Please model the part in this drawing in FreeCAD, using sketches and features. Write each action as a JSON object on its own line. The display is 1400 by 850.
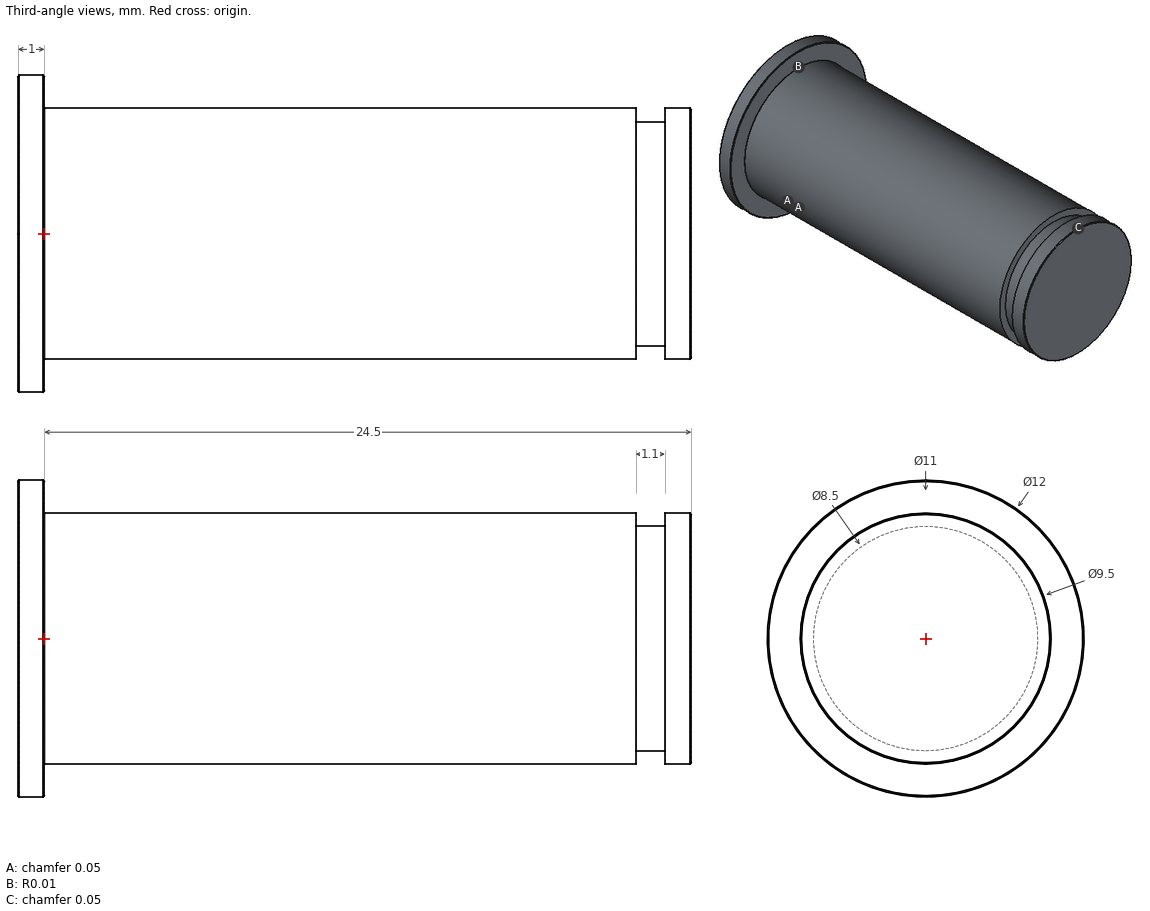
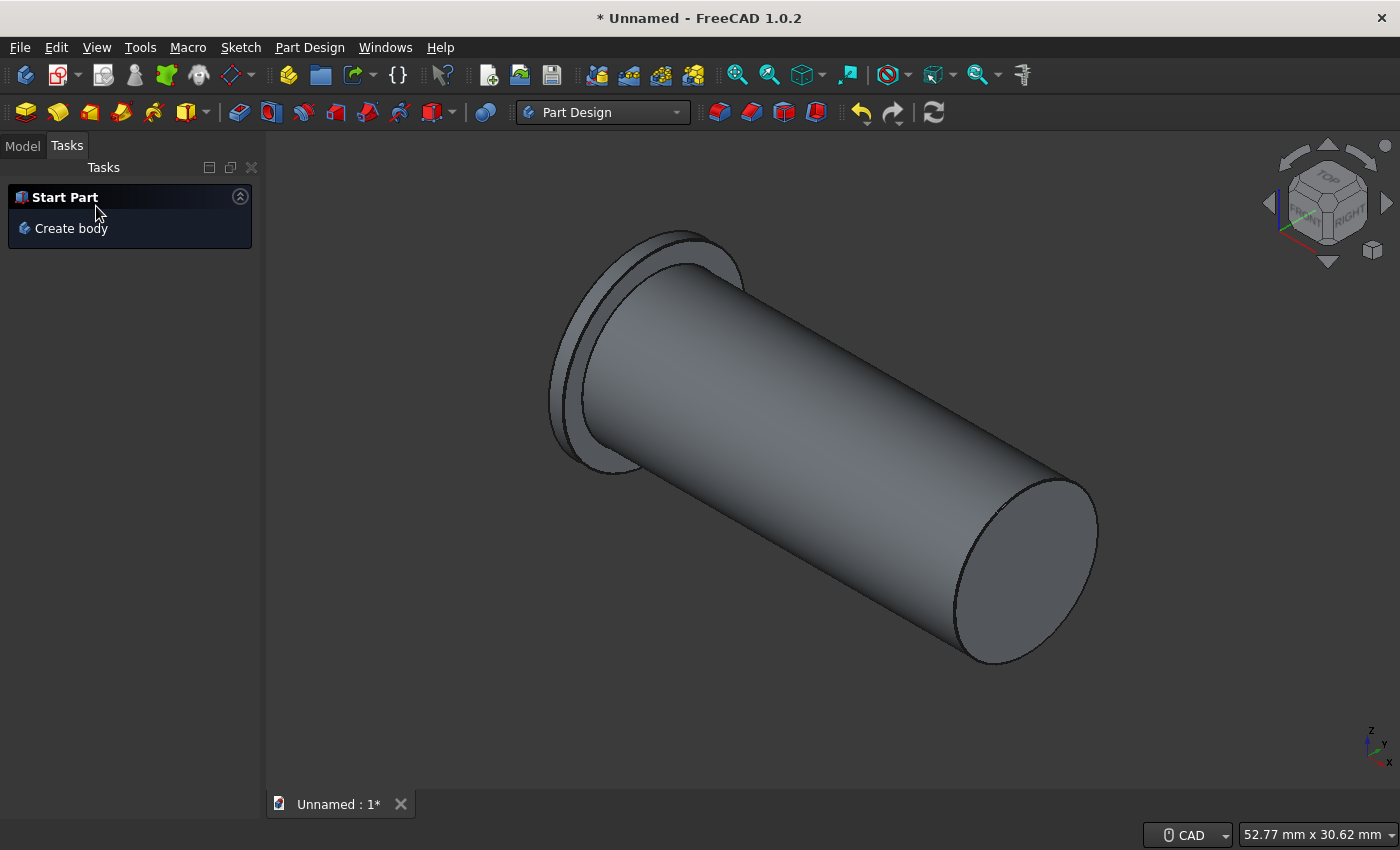
{"action": "left_click", "coordinate": [23, 145]}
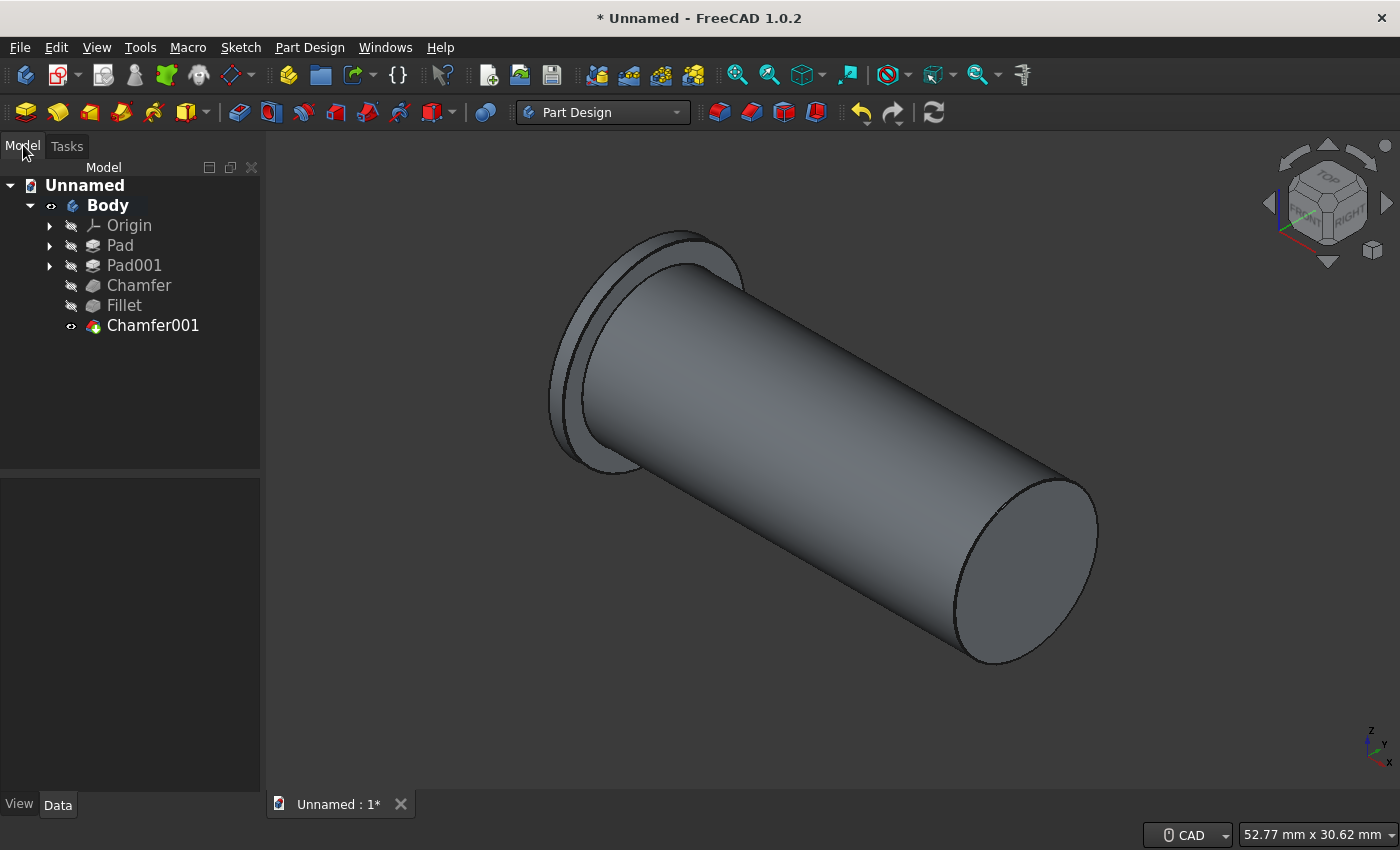
{"action": "left_click", "coordinate": [50, 226]}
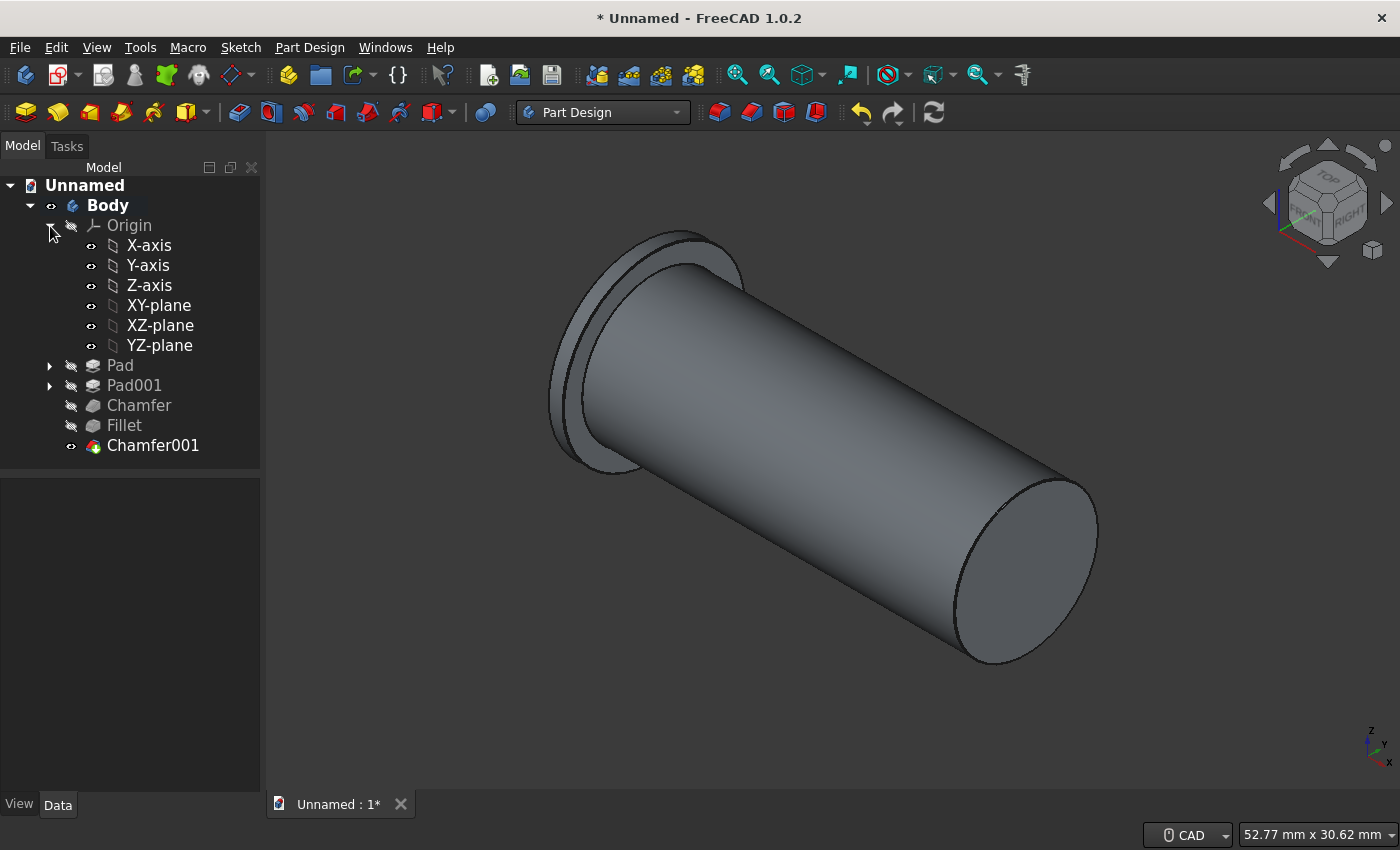
{"action": "left_click", "coordinate": [136, 346]}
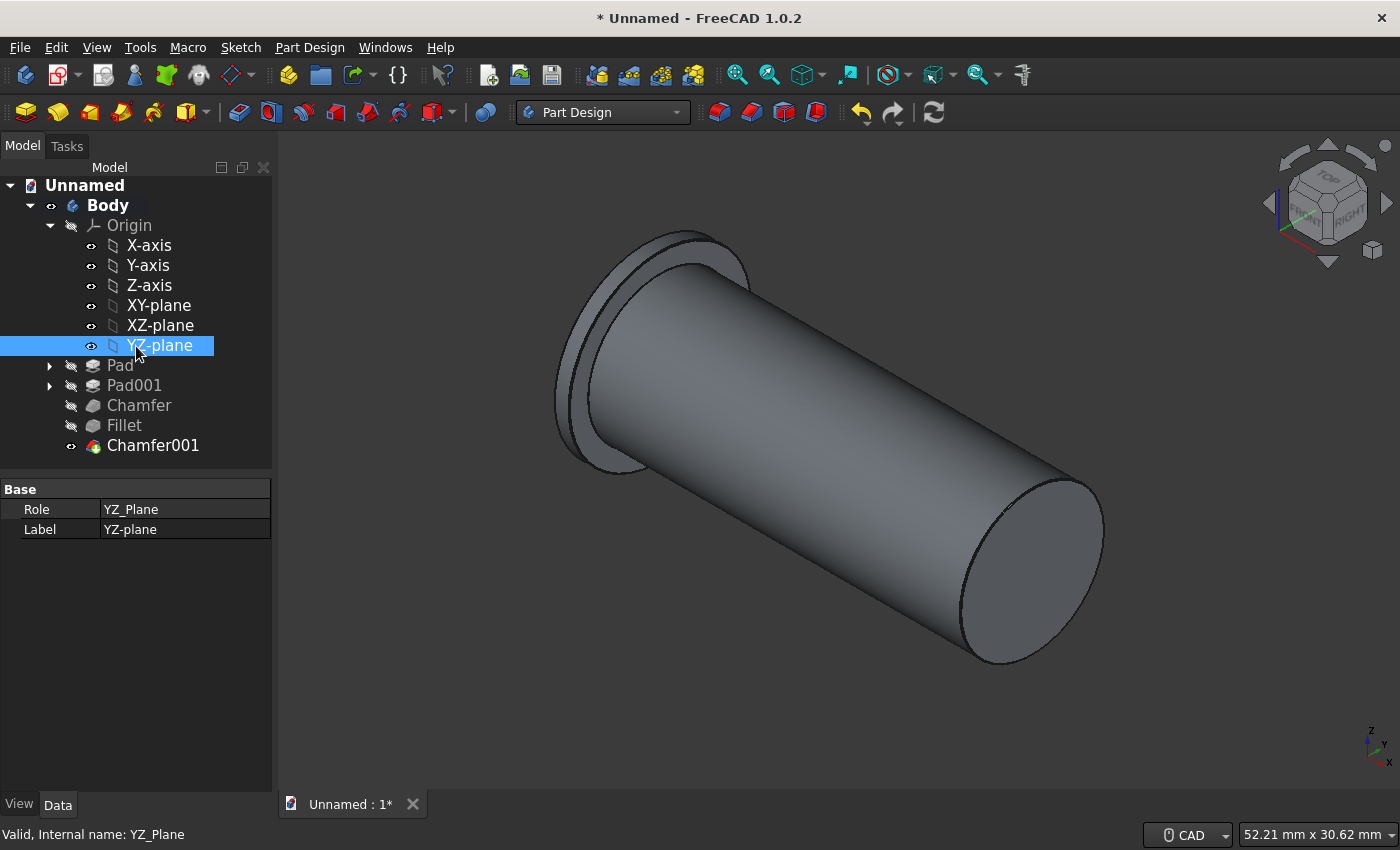
{"action": "left_click", "coordinate": [232, 76]}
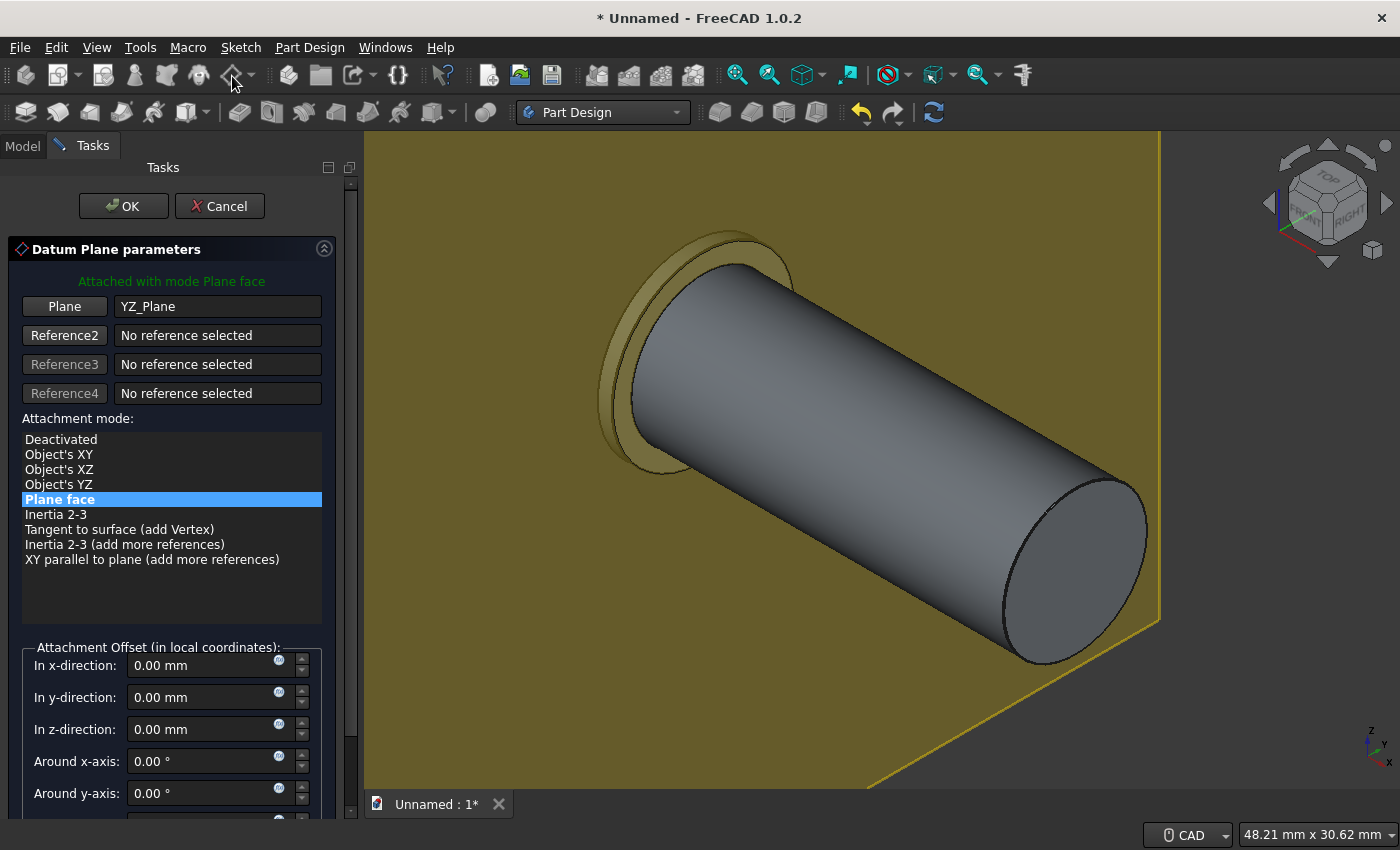
{"action": "triple_click", "coordinate": [210, 729]}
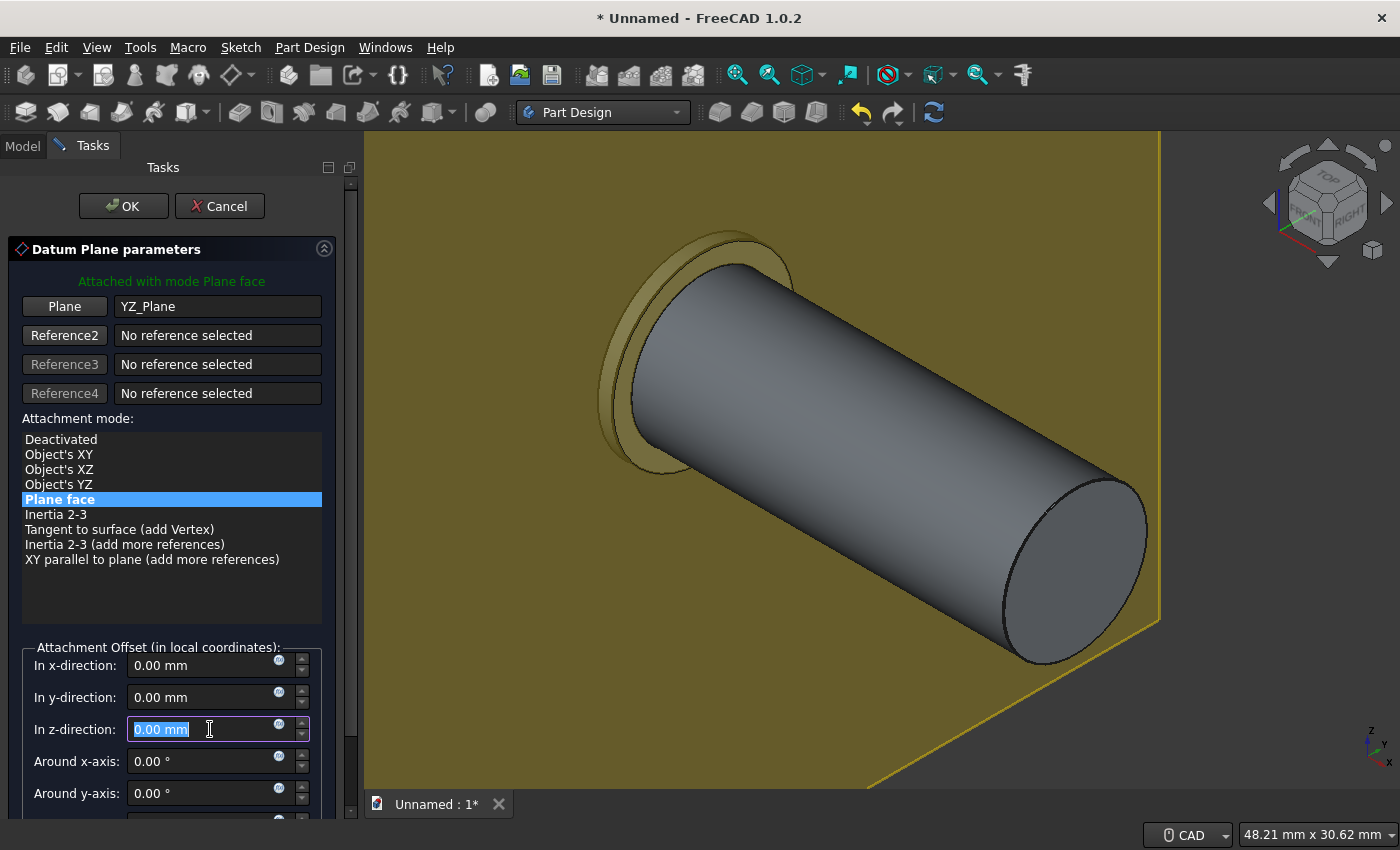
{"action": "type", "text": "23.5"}
{"action": "key", "text": "Tab"}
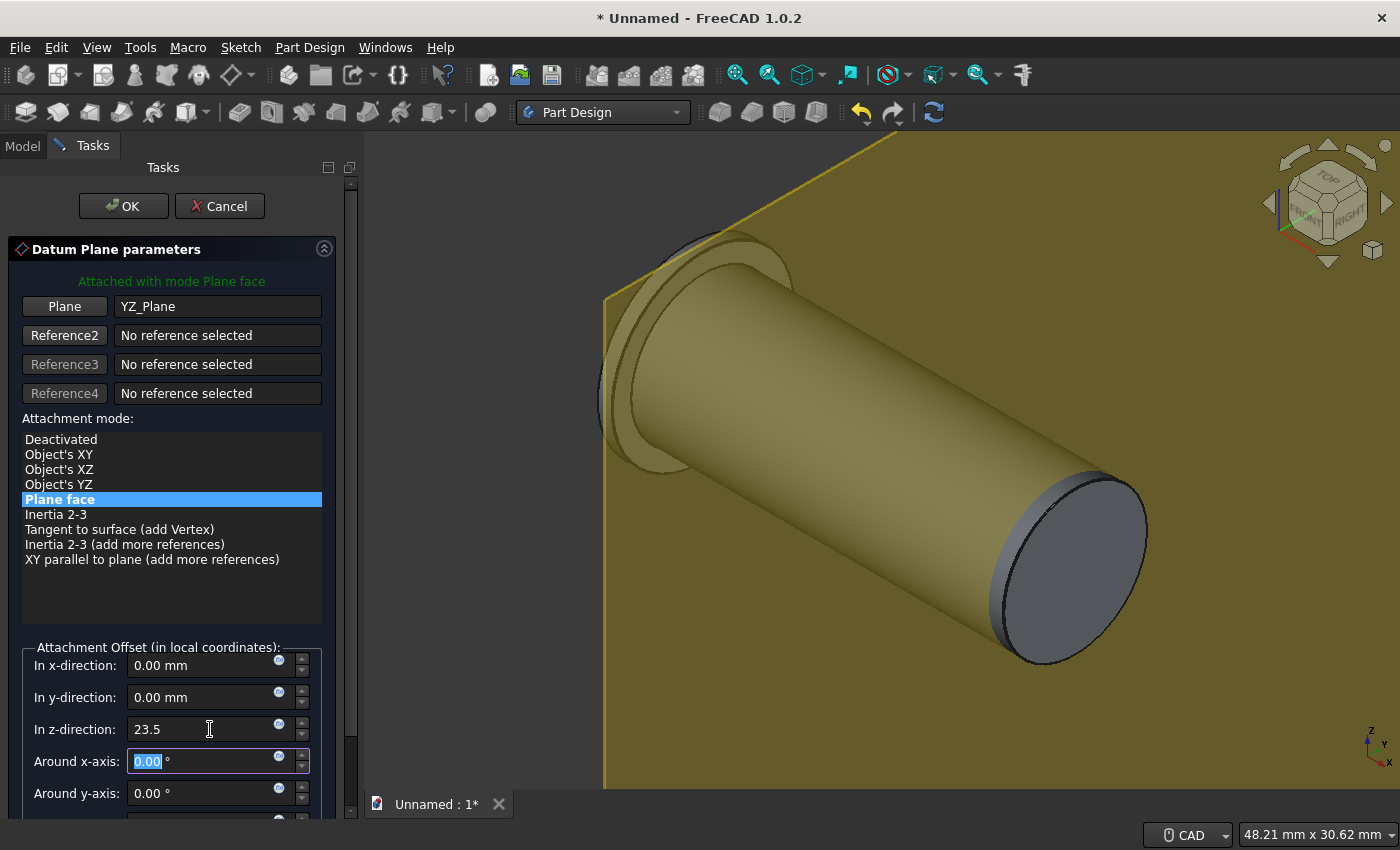
{"action": "left_click", "coordinate": [124, 206]}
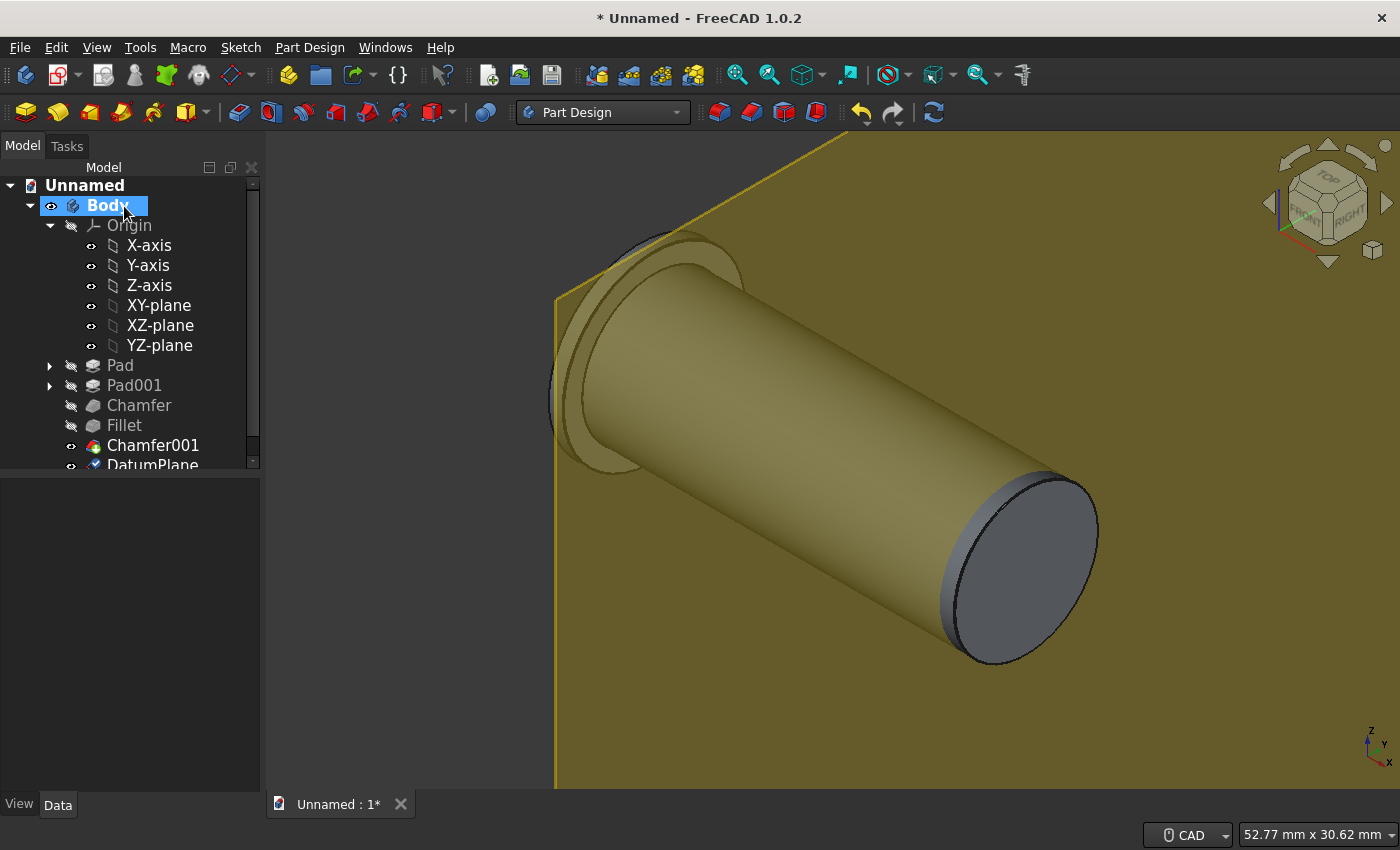
{"action": "left_click", "coordinate": [116, 466]}